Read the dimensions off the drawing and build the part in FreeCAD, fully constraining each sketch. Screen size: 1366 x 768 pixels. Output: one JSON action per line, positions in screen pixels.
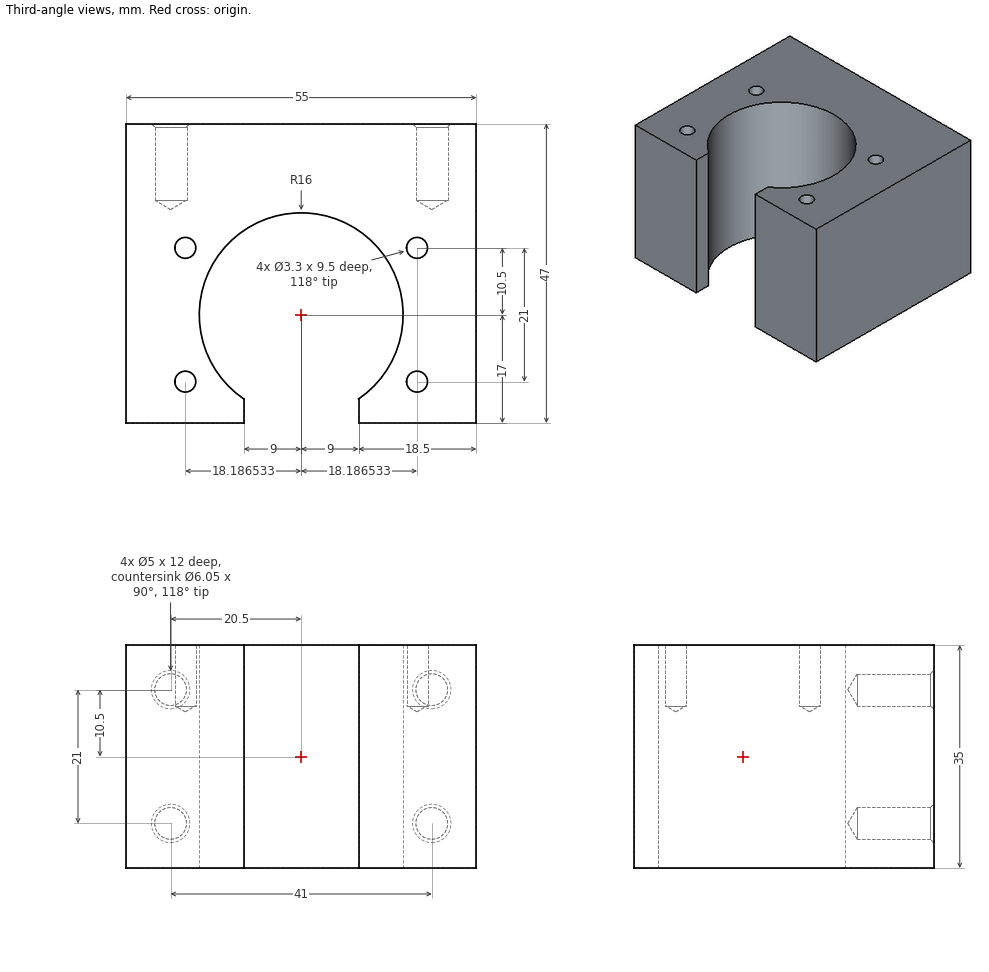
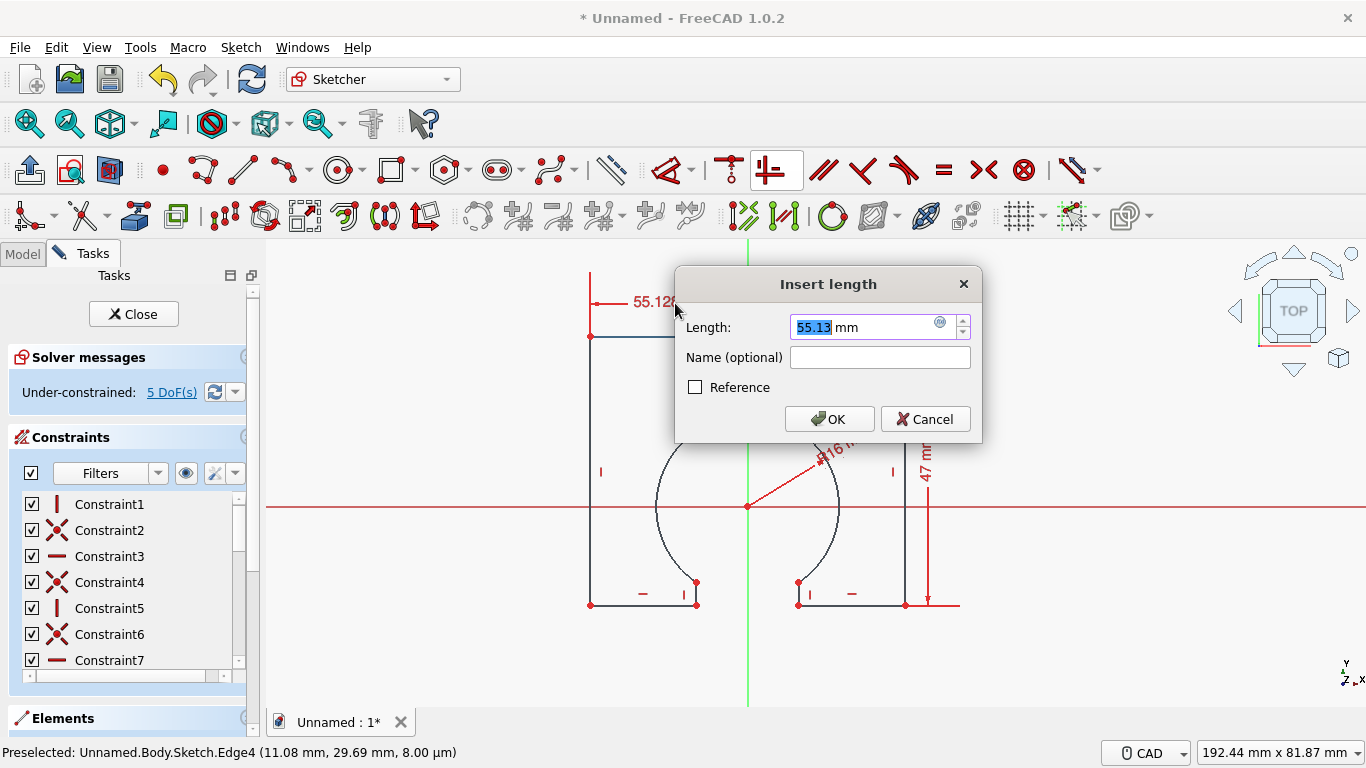
{"action": "type", "text": "55"}
{"action": "key", "text": "Return"}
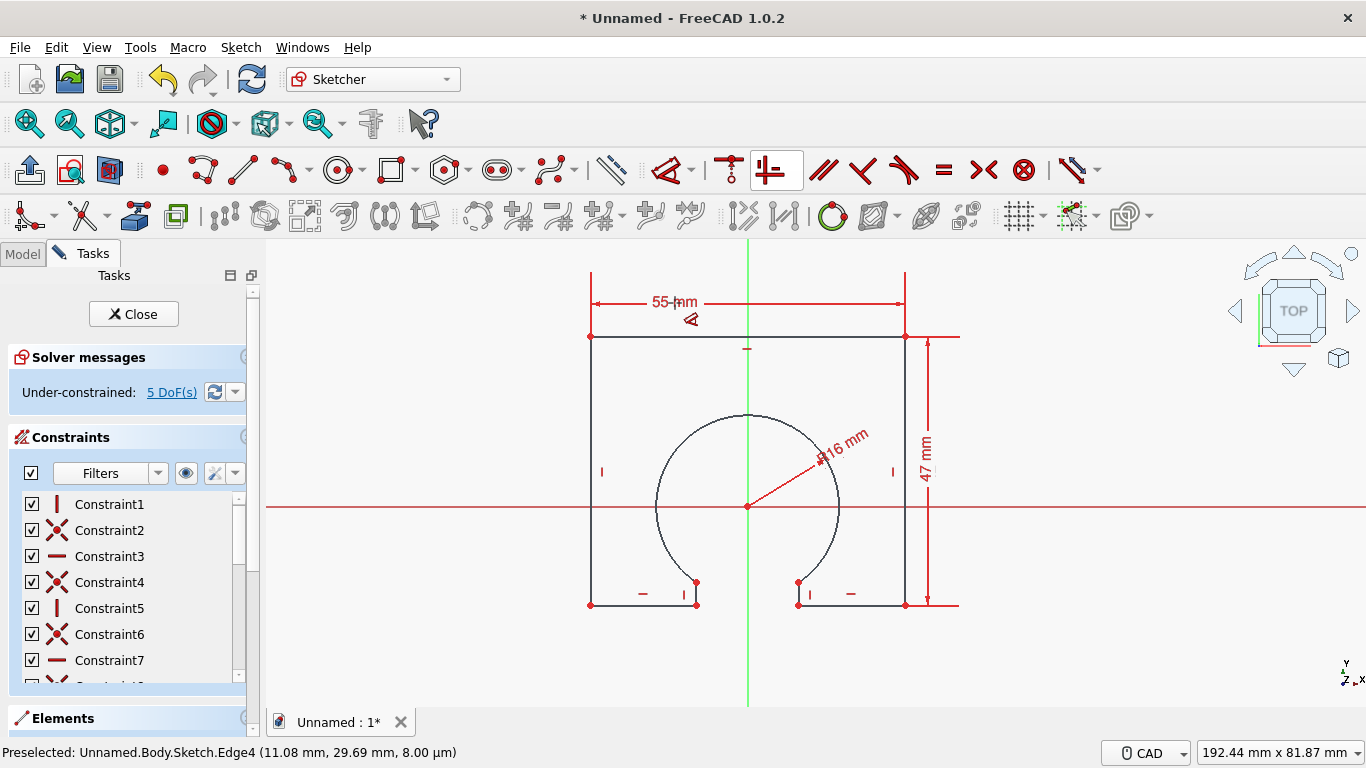
{"action": "left_click", "coordinate": [591, 418]}
{"action": "left_click", "coordinate": [557, 471]}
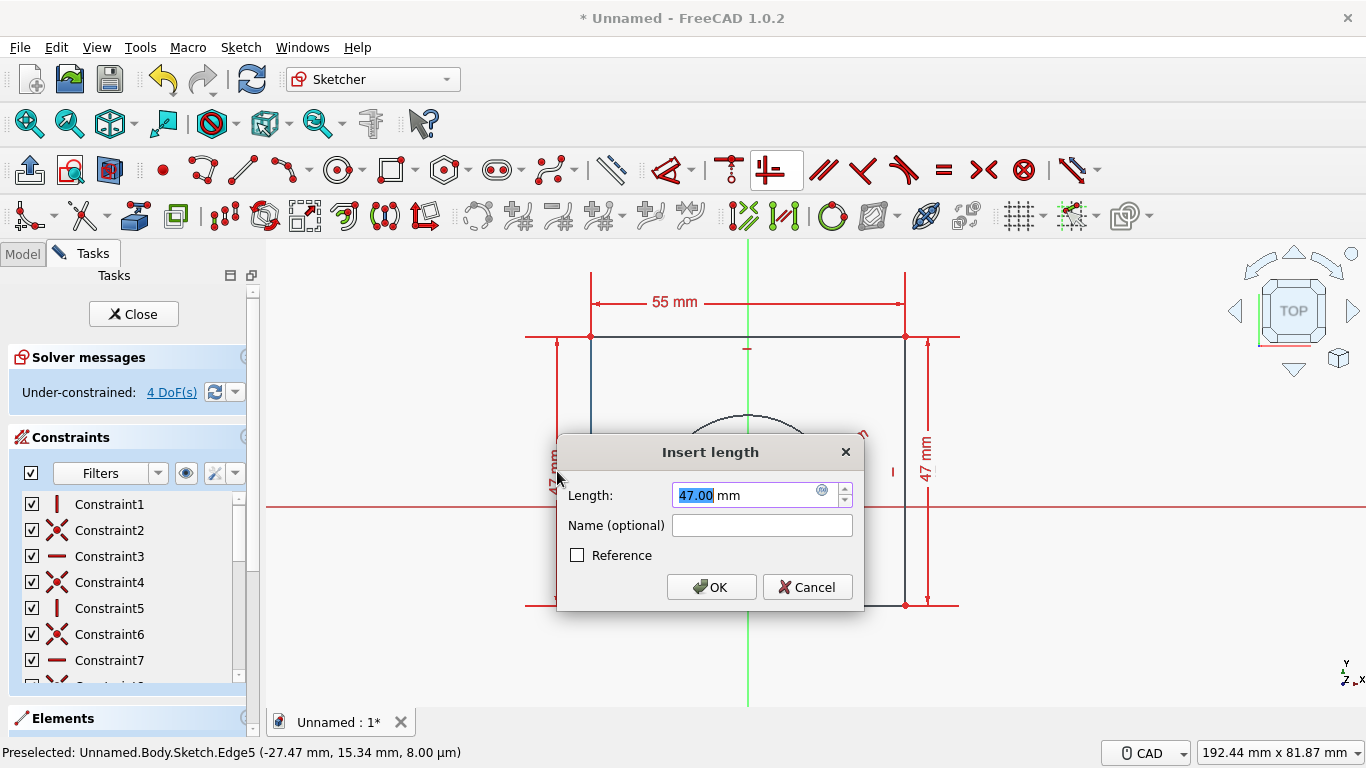
{"action": "type", "text": "47"}
{"action": "key", "text": "Return"}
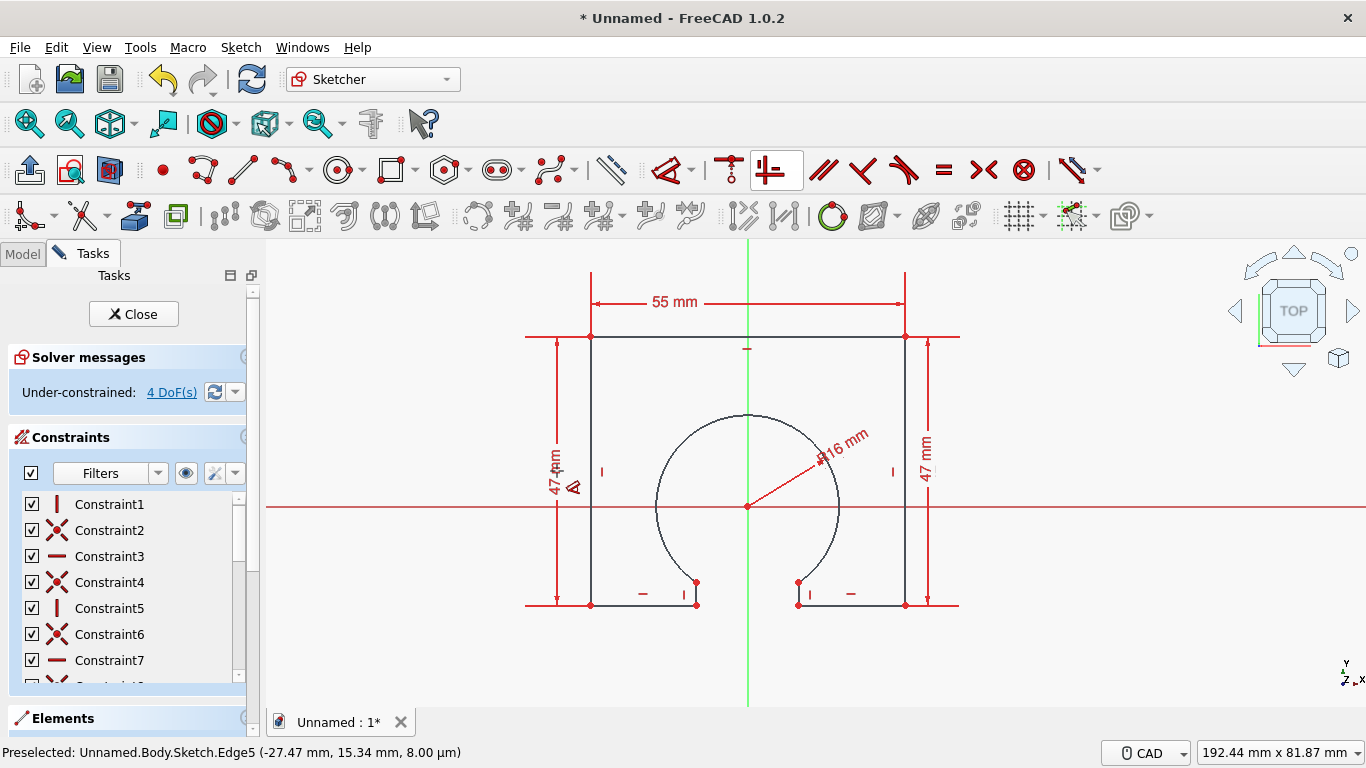
{"action": "left_click", "coordinate": [799, 582]}
{"action": "left_click", "coordinate": [773, 616]}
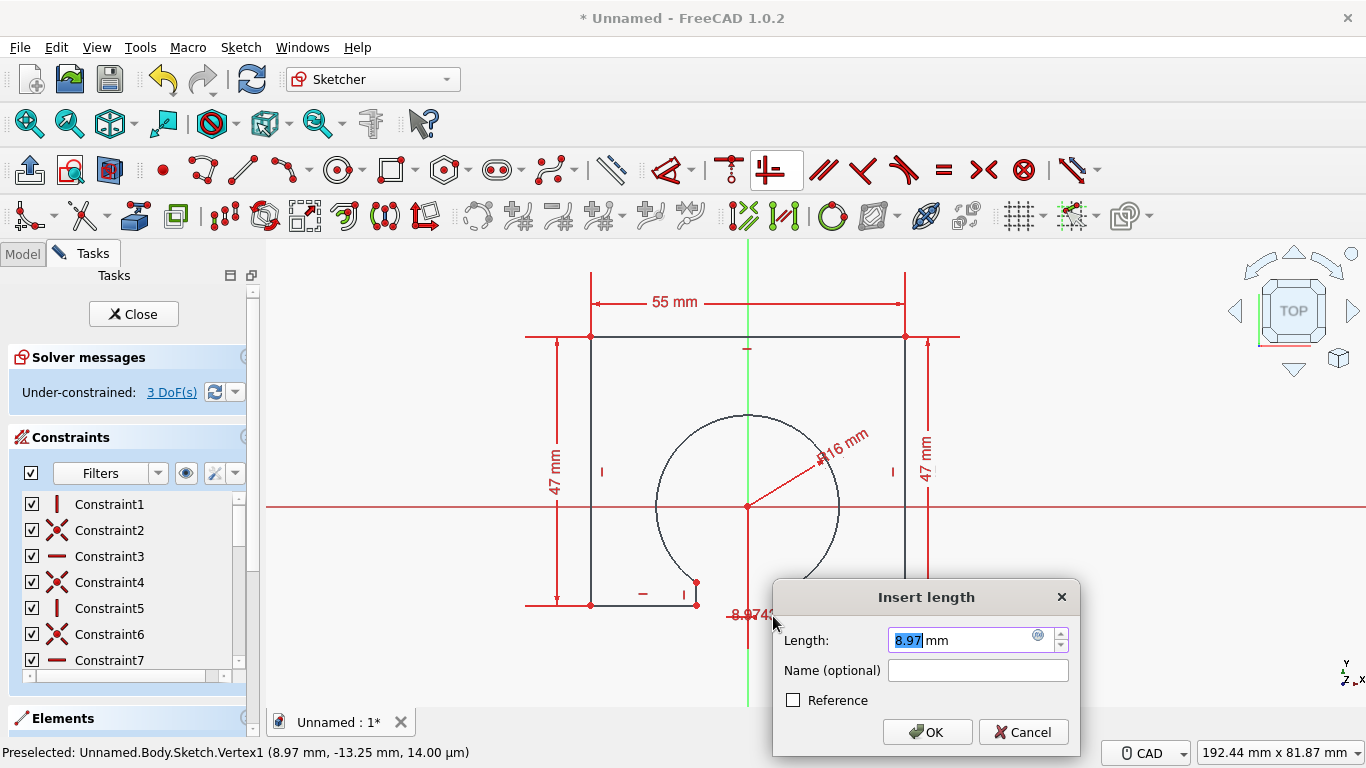
{"action": "type", "text": "9"}
{"action": "key", "text": "Return"}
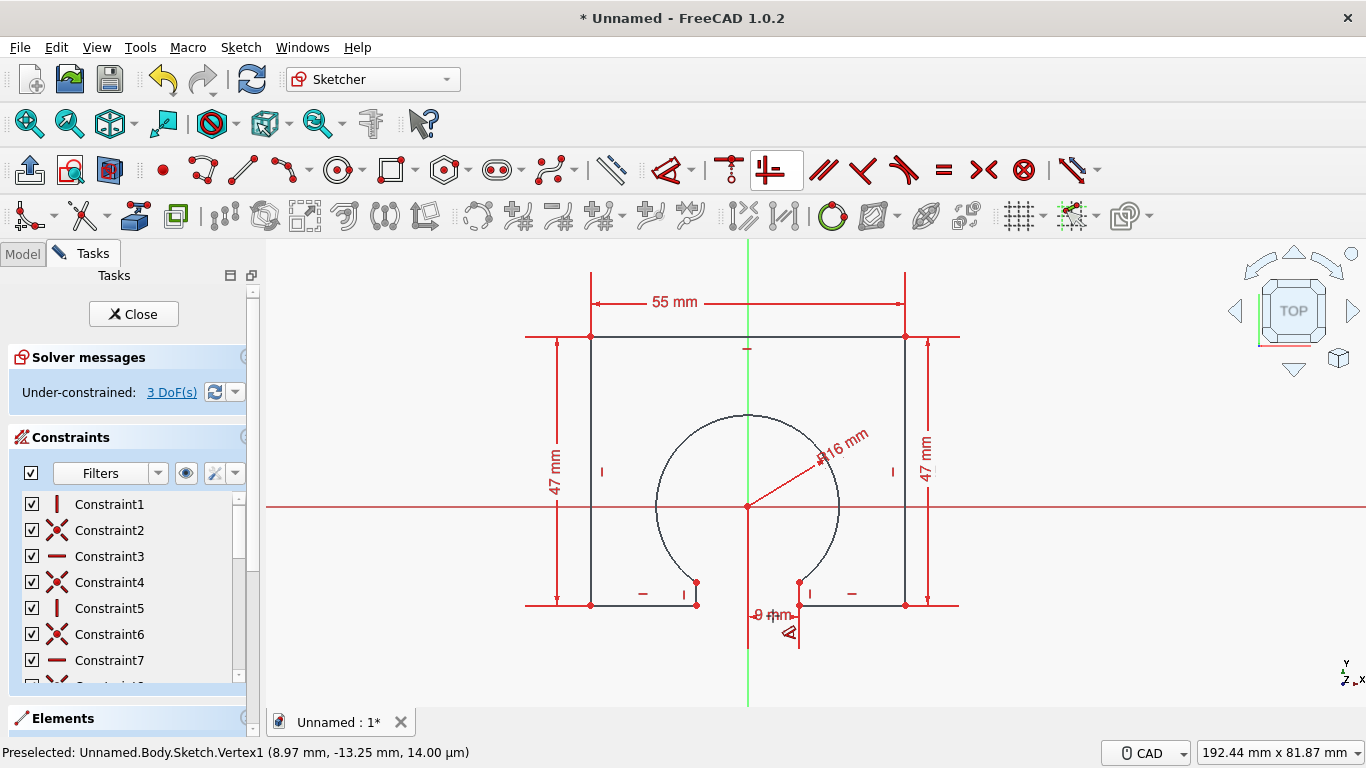
{"action": "left_click", "coordinate": [696, 606]}
{"action": "left_click", "coordinate": [722, 640]}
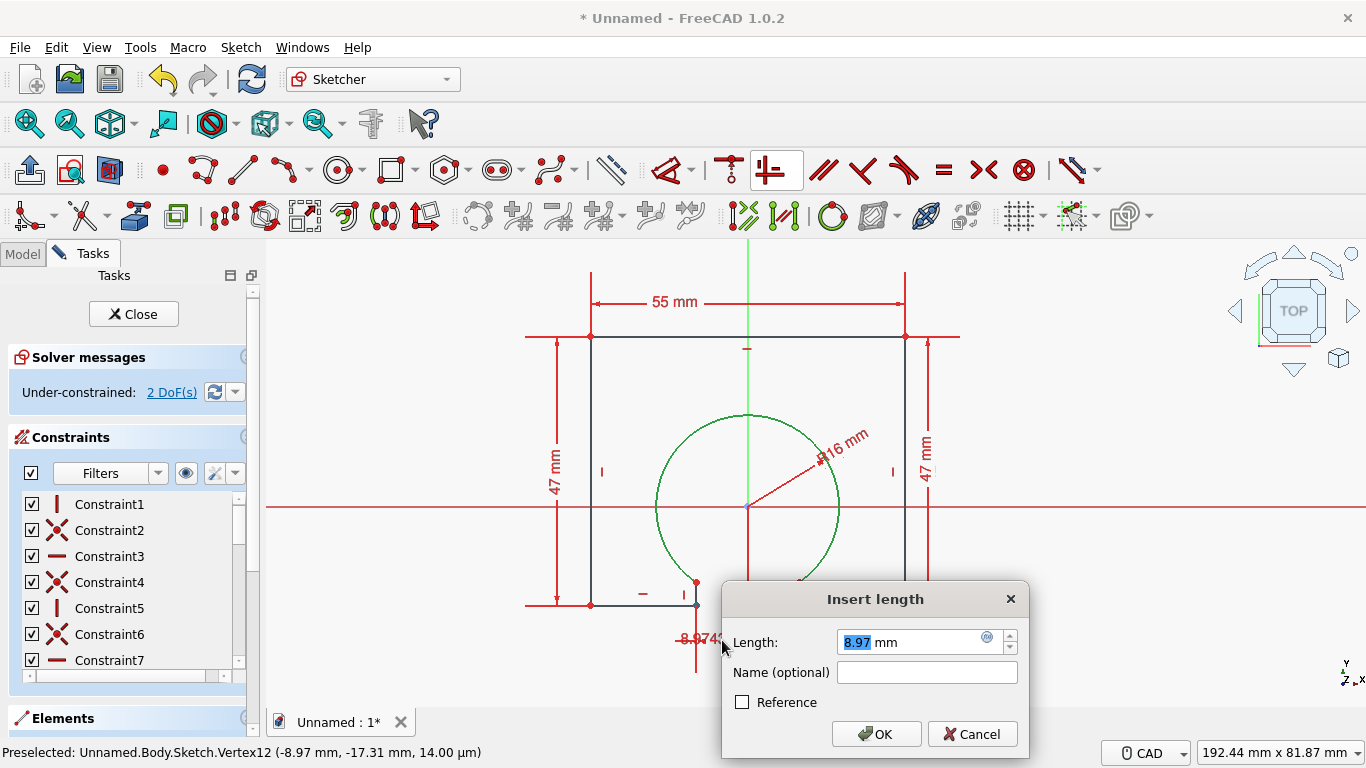
{"action": "type", "text": "9"}
{"action": "key", "text": "Return"}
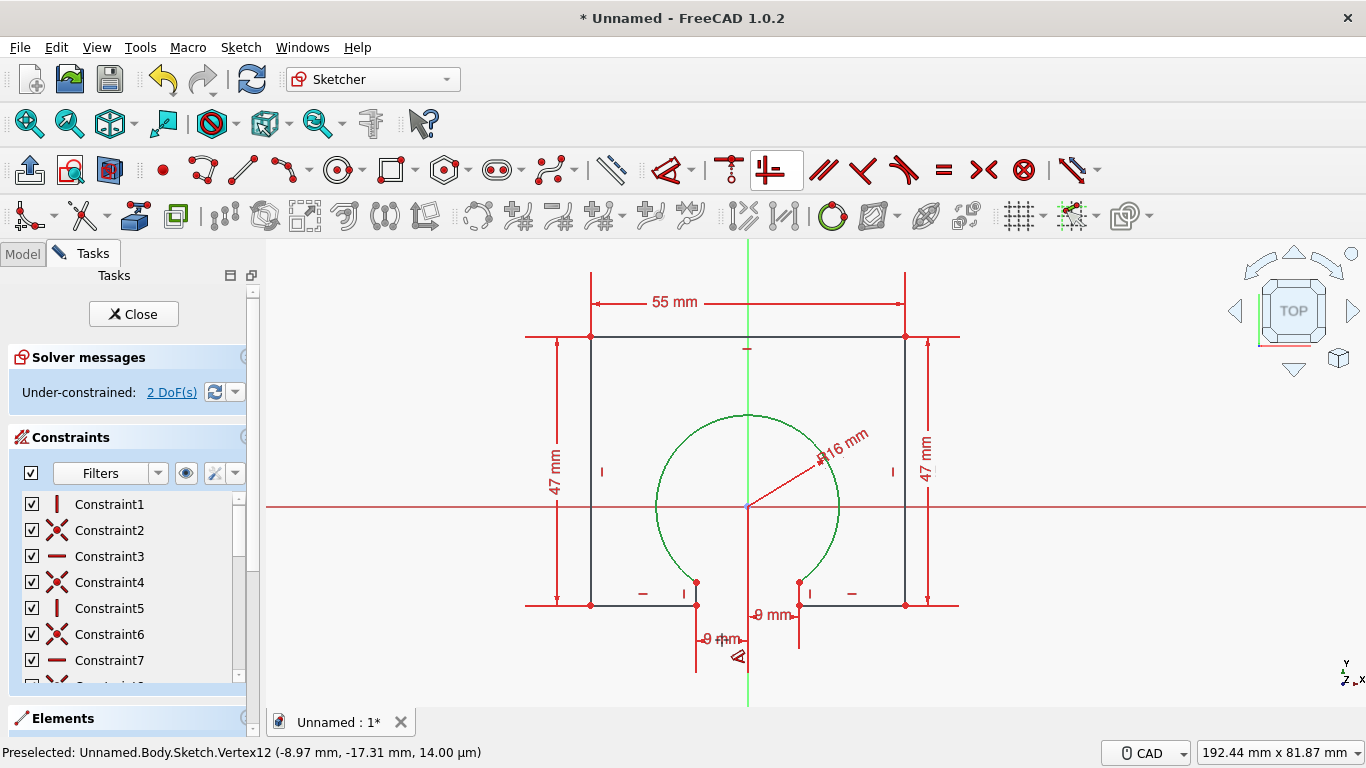
{"action": "left_click", "coordinate": [799, 606]}
{"action": "left_click", "coordinate": [833, 579]}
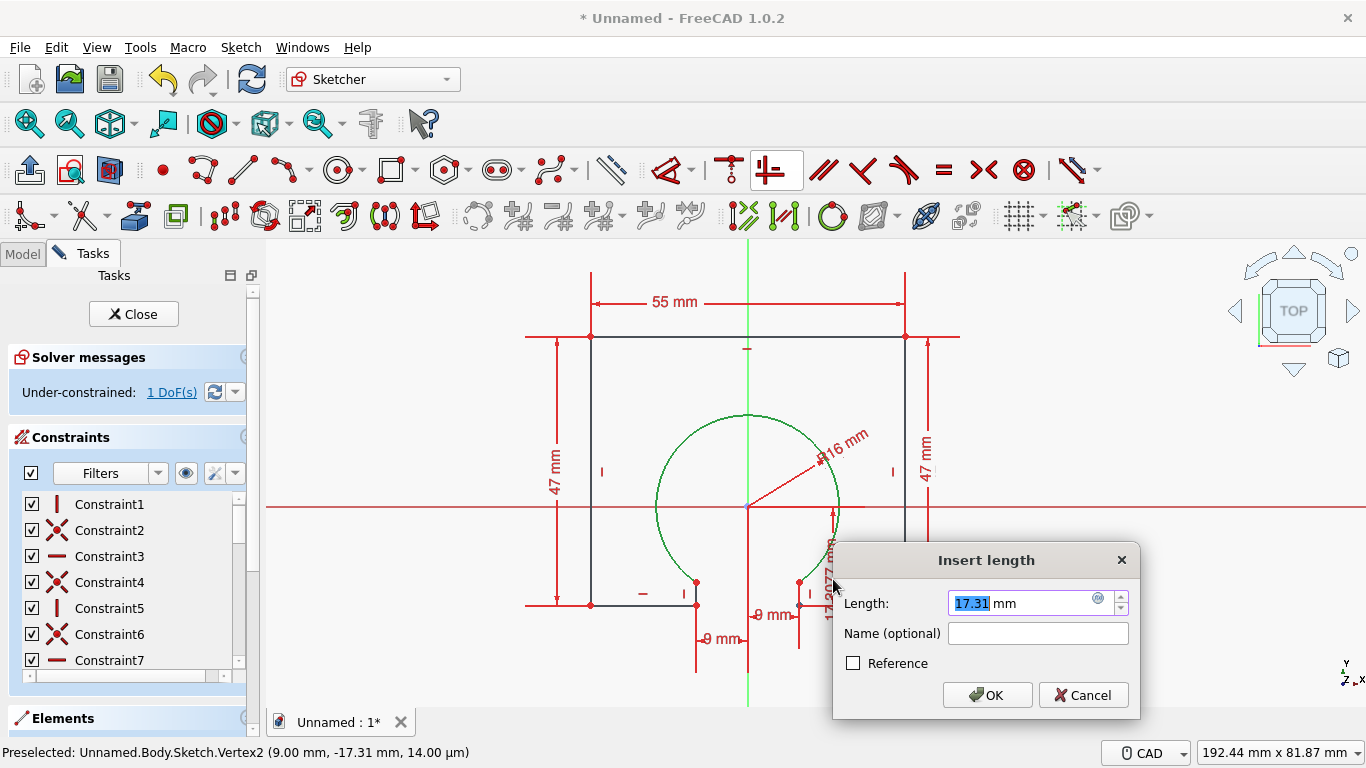
{"action": "type", "text": "17"}
{"action": "key", "text": "Return"}